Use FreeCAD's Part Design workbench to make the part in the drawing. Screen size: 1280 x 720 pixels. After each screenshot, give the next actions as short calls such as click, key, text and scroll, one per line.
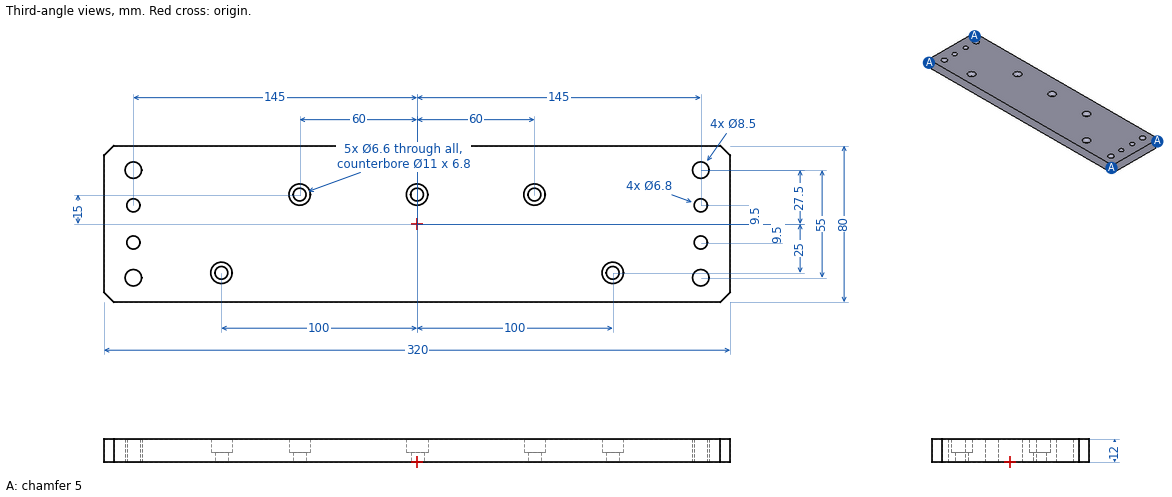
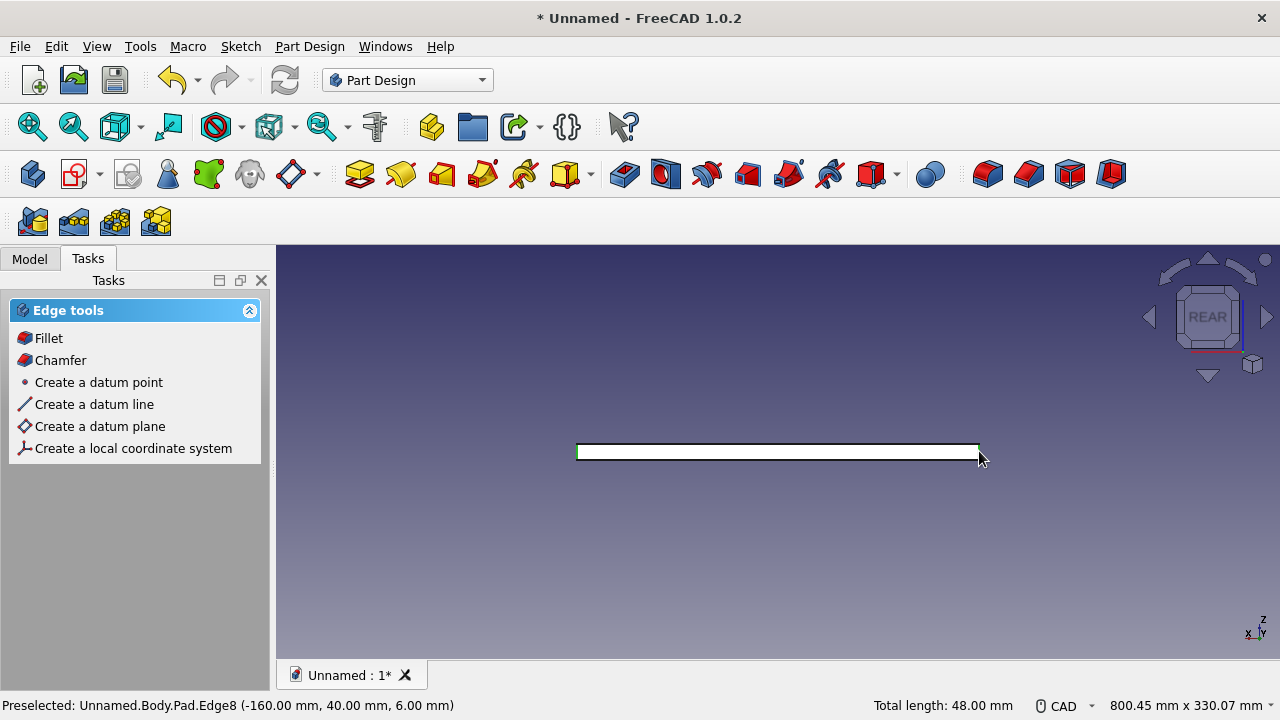
click(1029, 174)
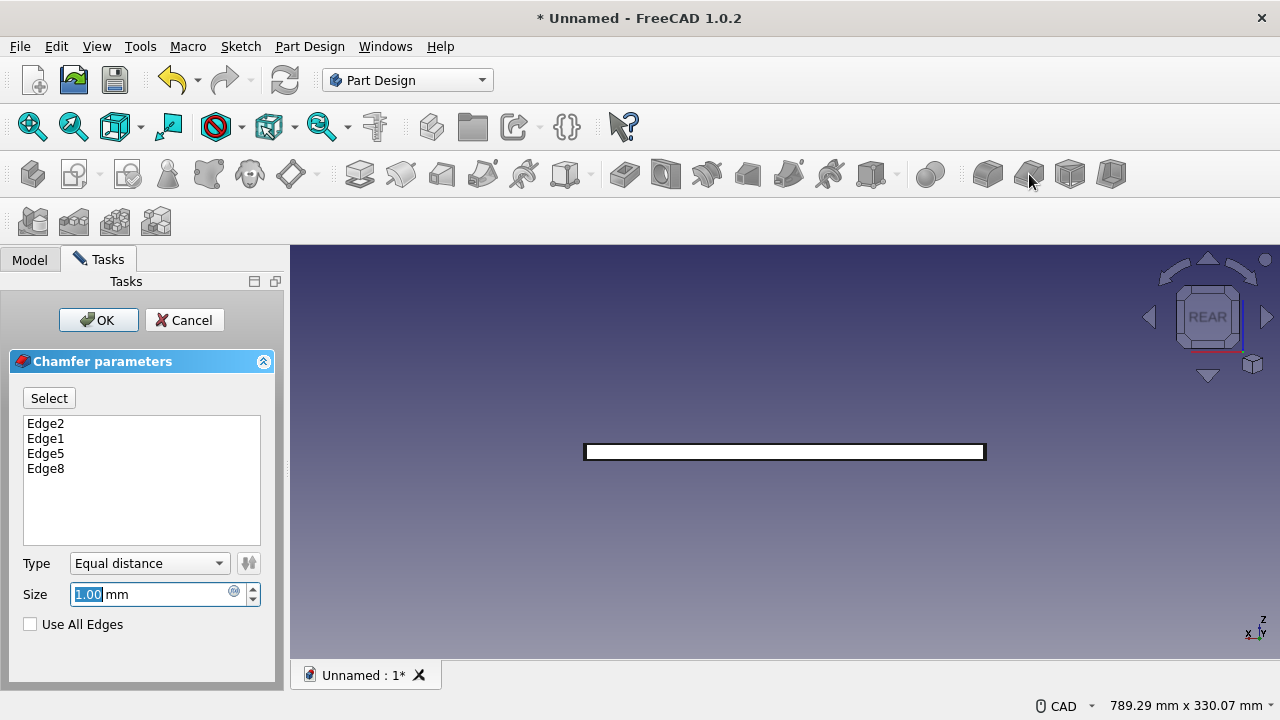
text(5)
key(Tab)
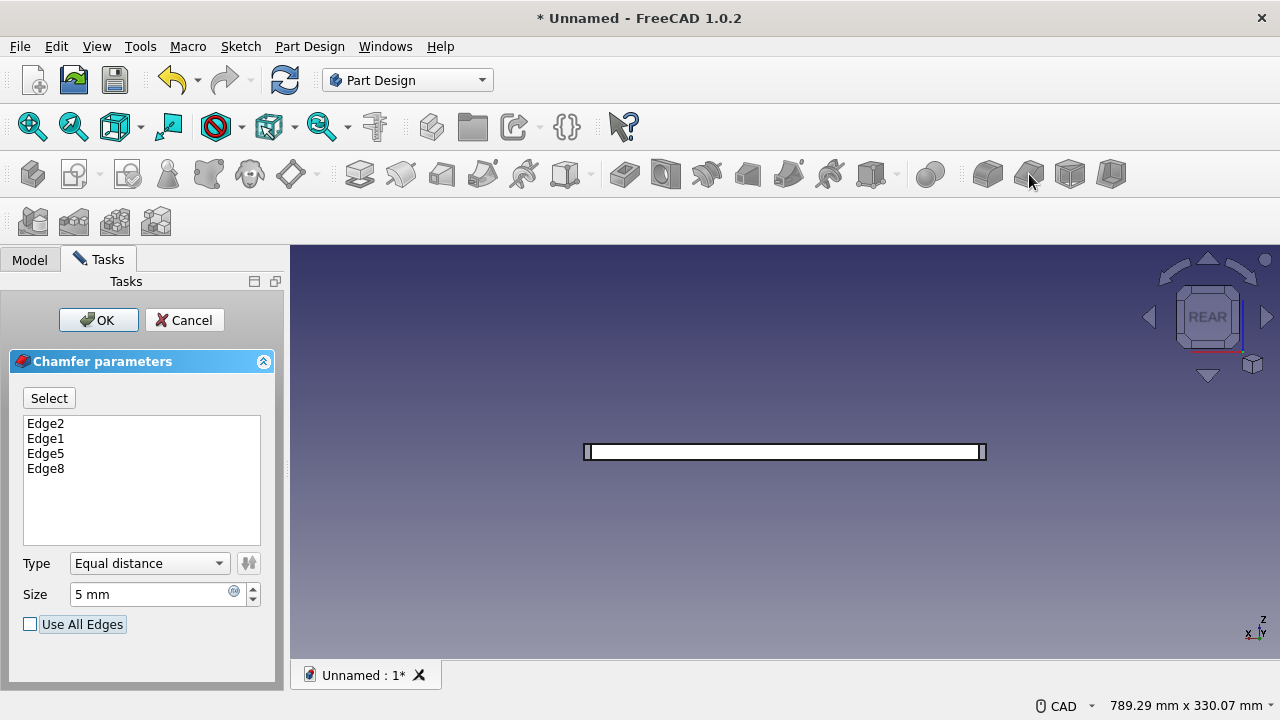
click(99, 320)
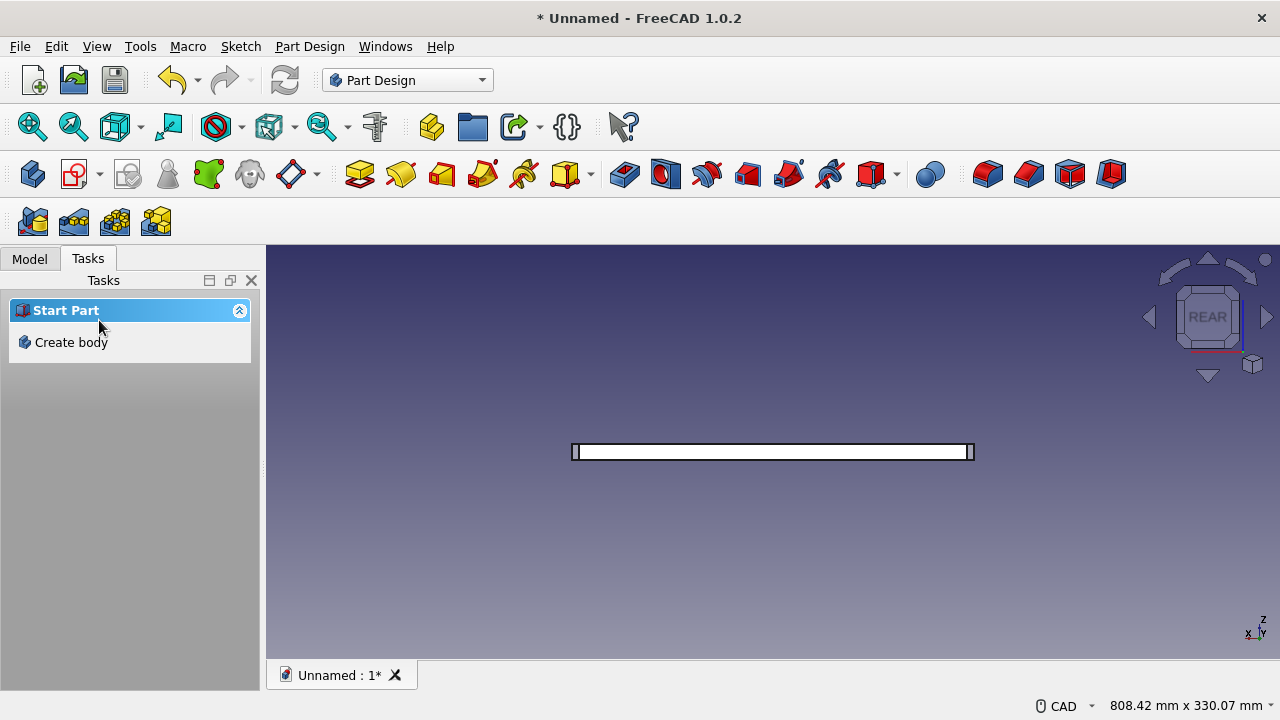
click(33, 128)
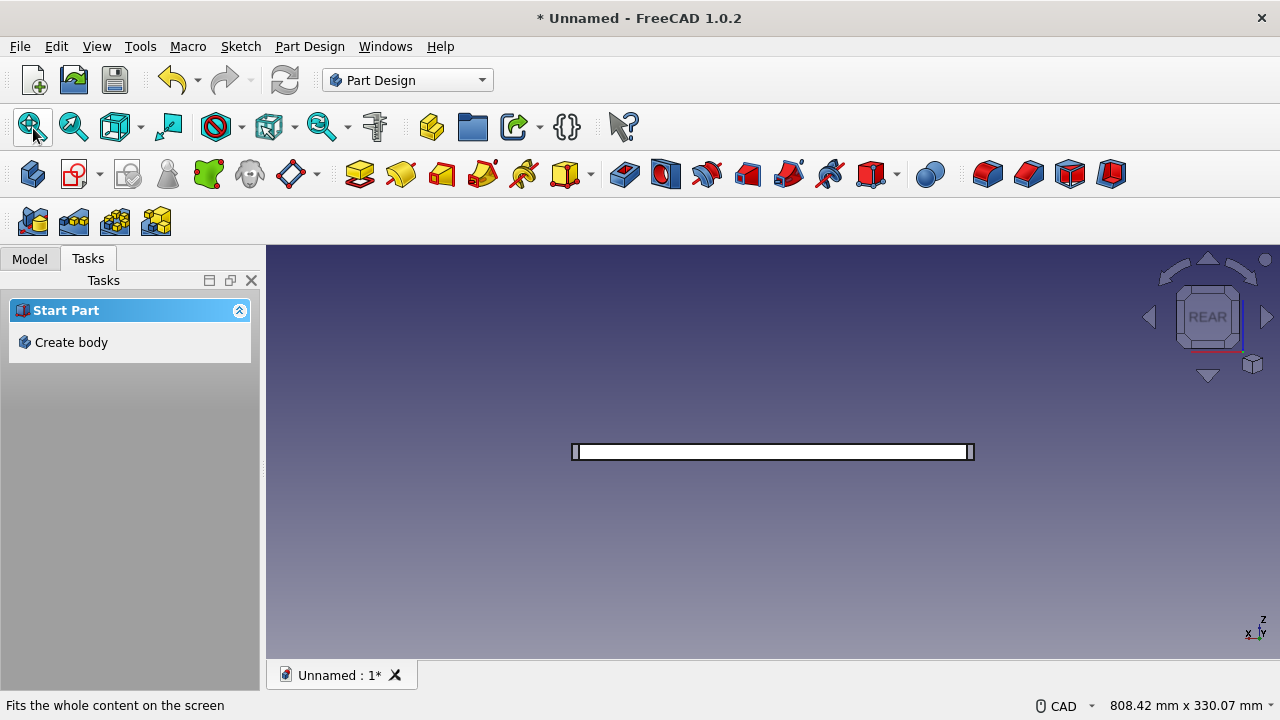
click(74, 174)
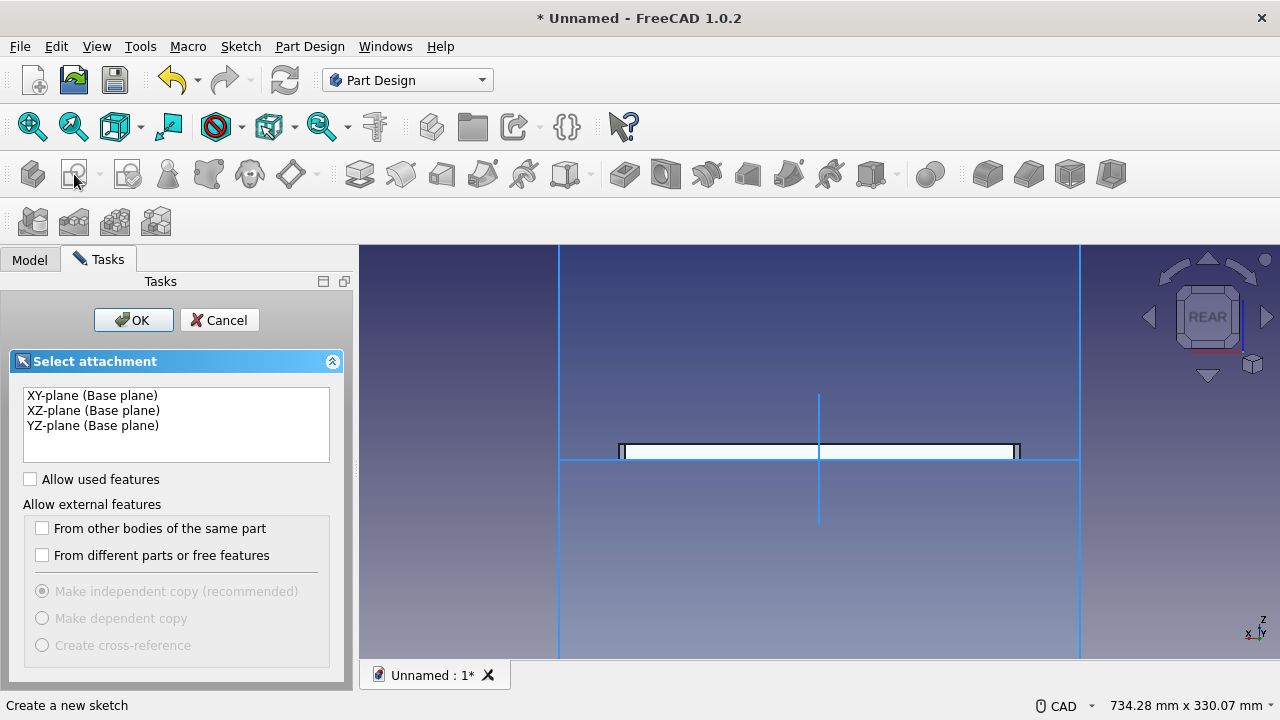
click(84, 396)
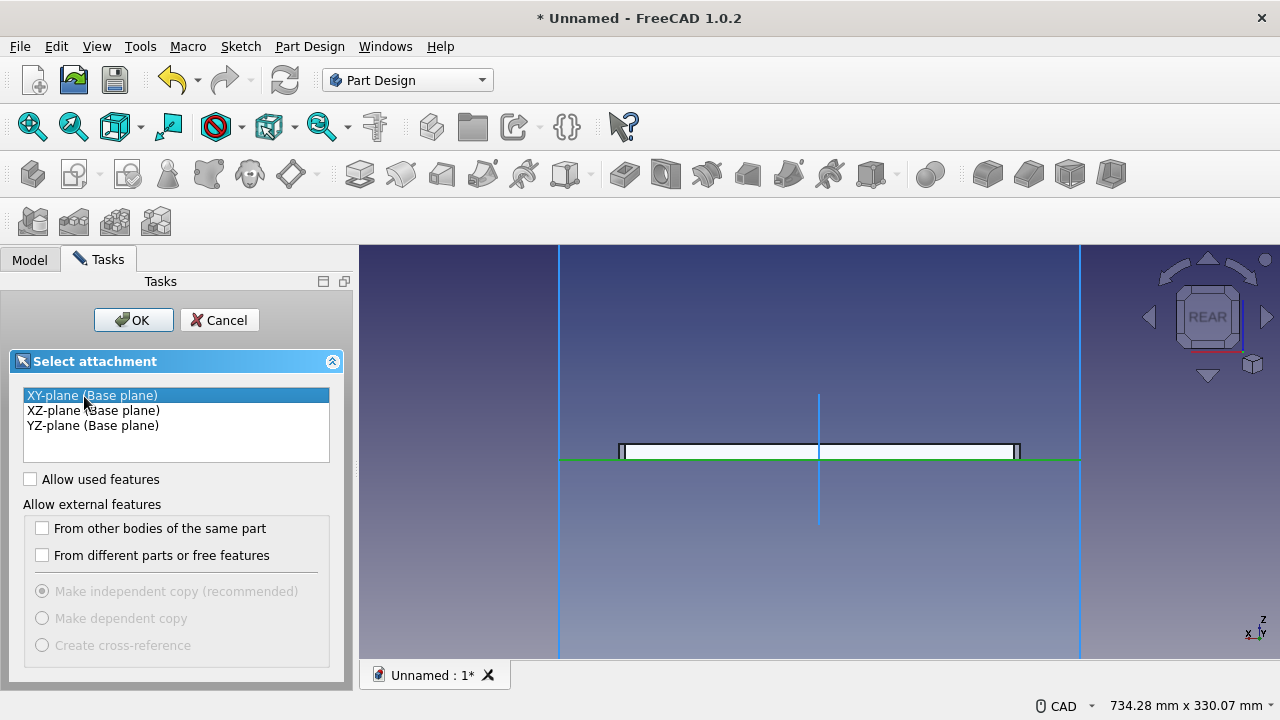
click(134, 320)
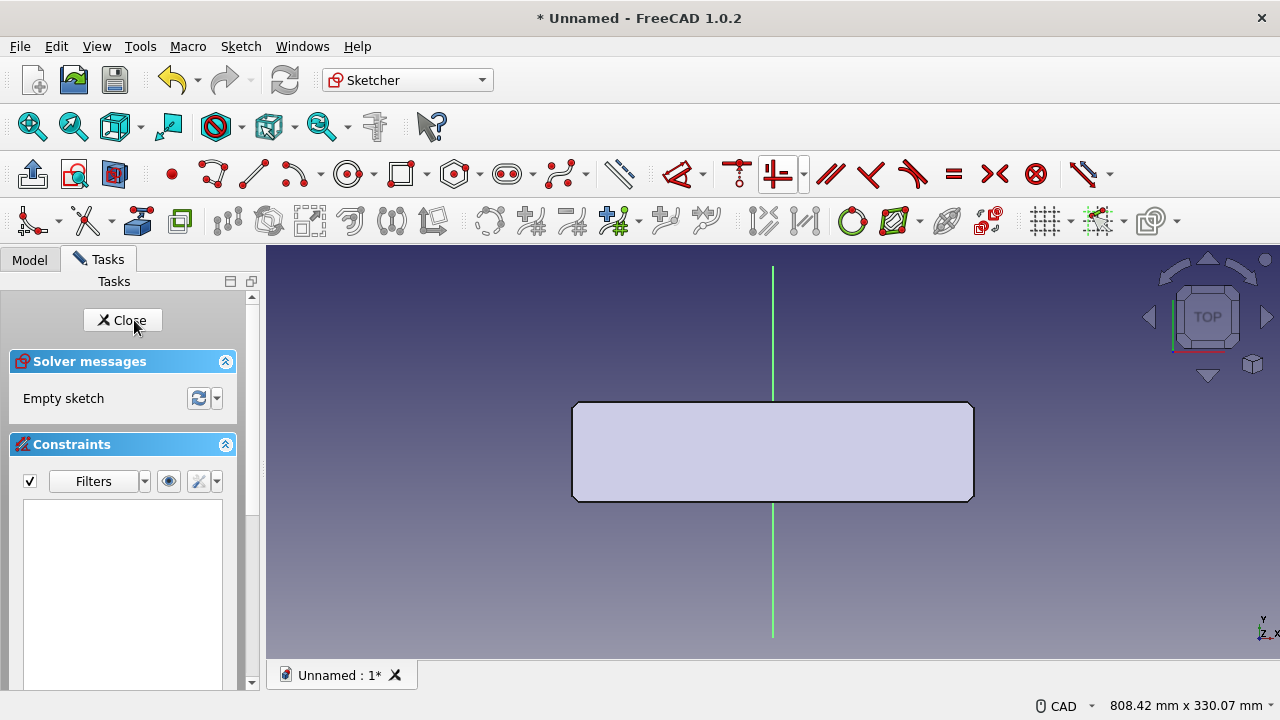
key(q)
key(s)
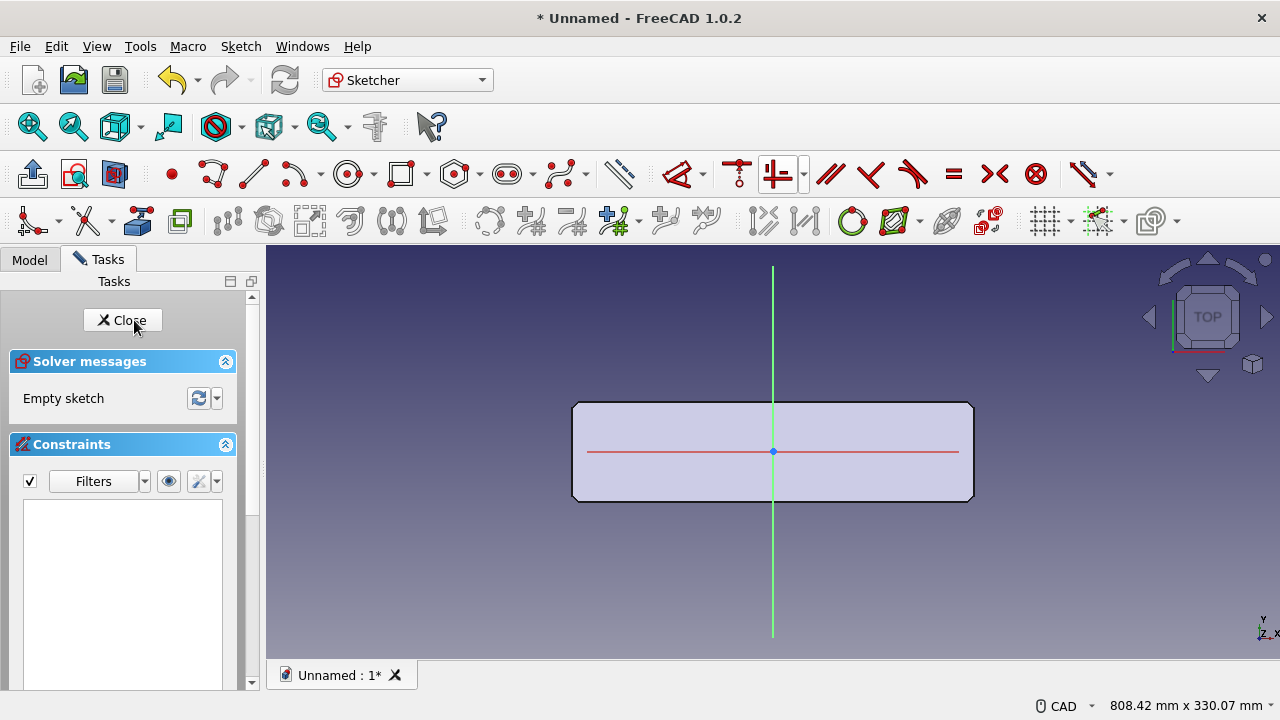
scroll(912, 452, up, 2)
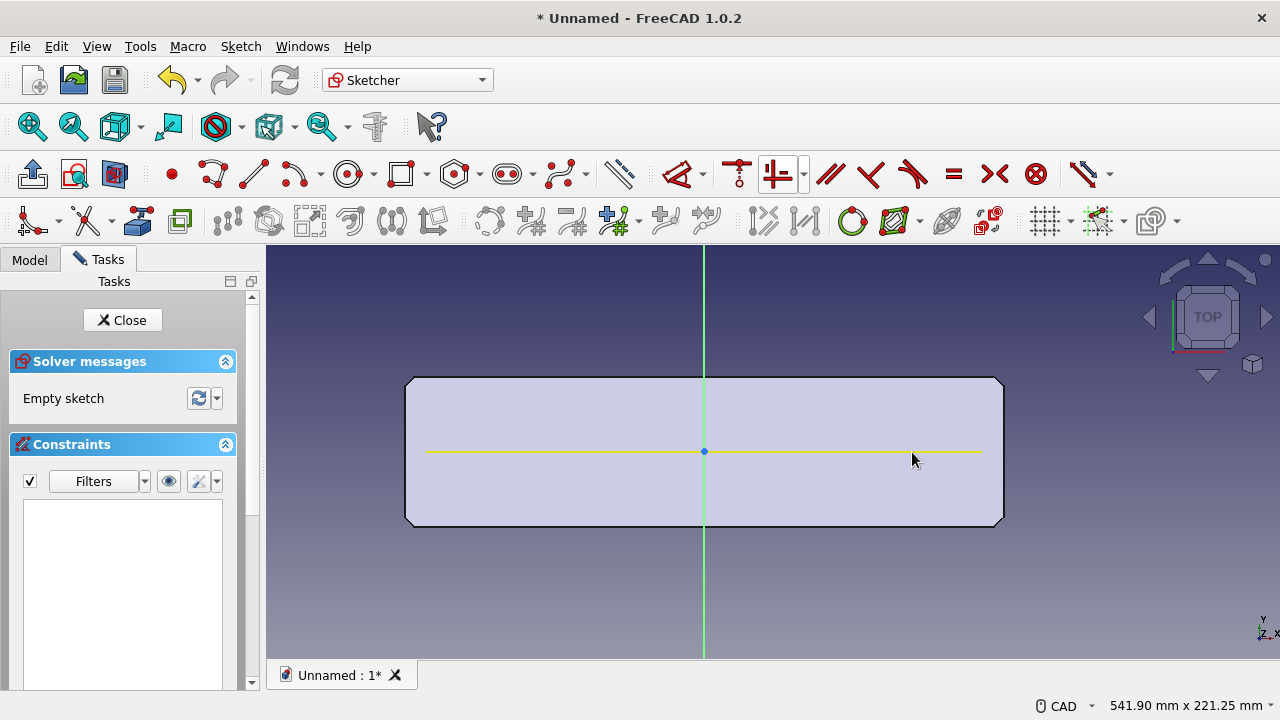
click(348, 174)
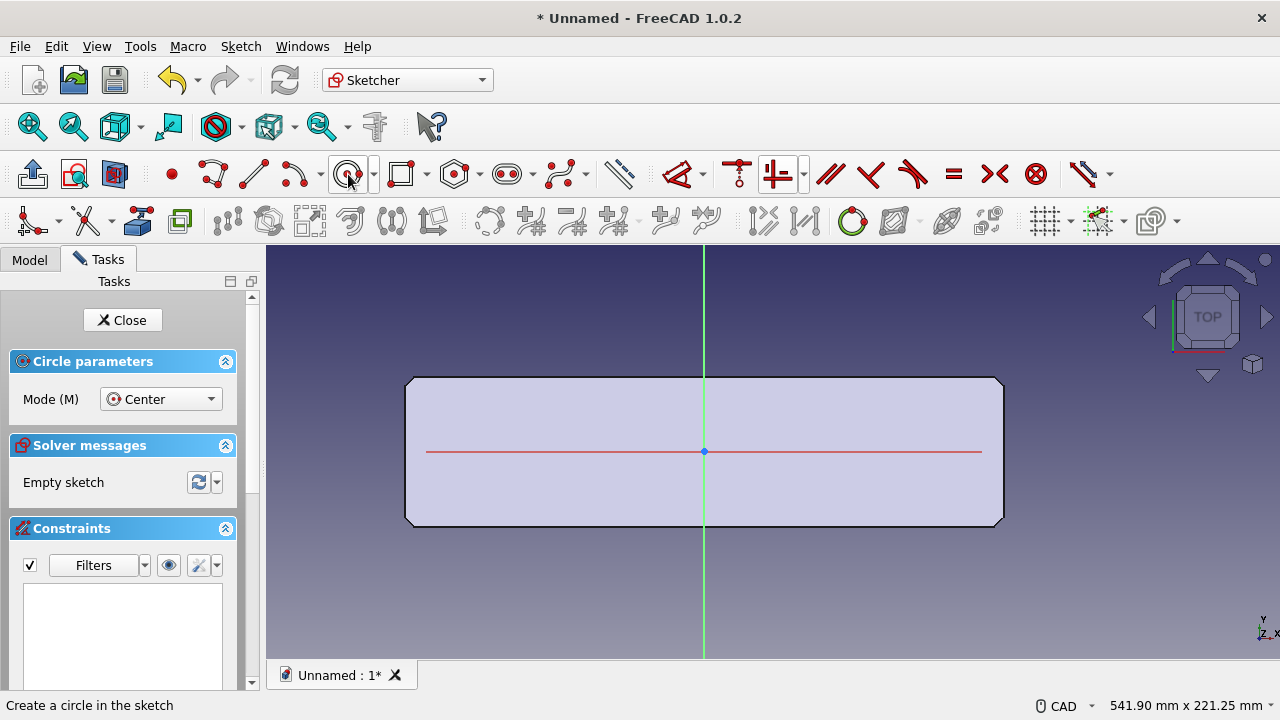
scroll(976, 434, up, 7)